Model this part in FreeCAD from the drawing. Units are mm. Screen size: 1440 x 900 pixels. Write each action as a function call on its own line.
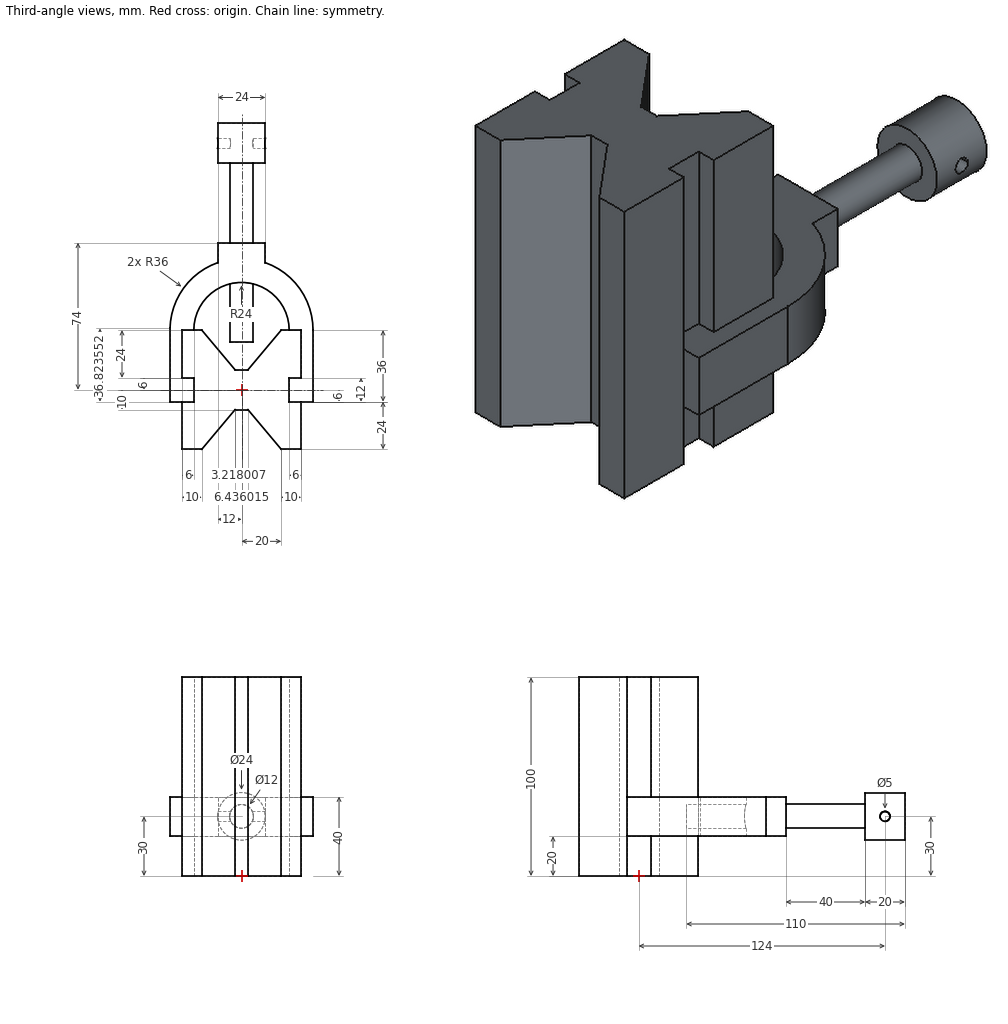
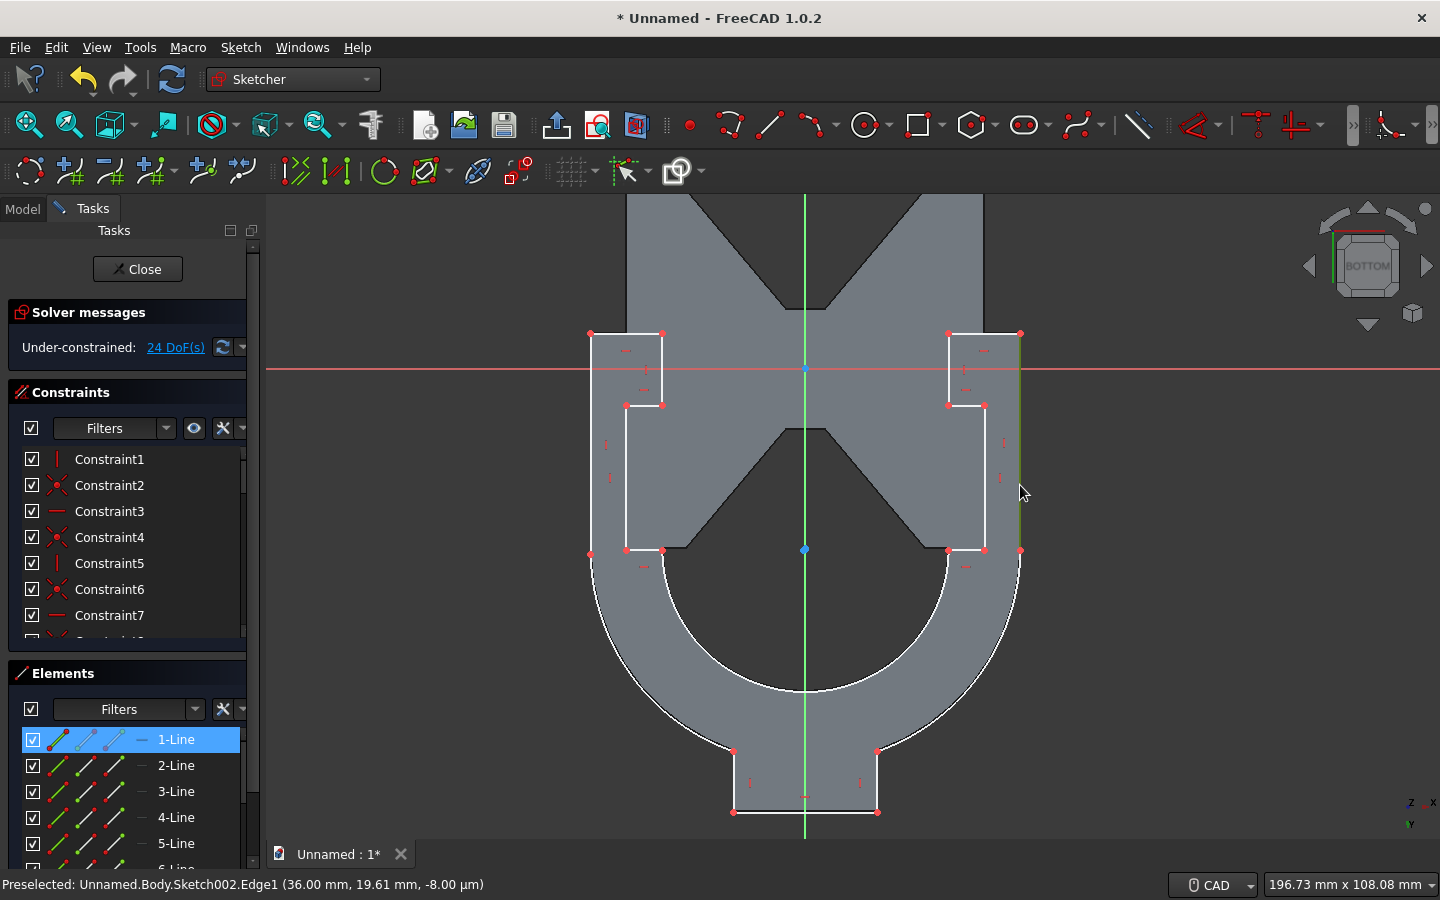
click(945, 712)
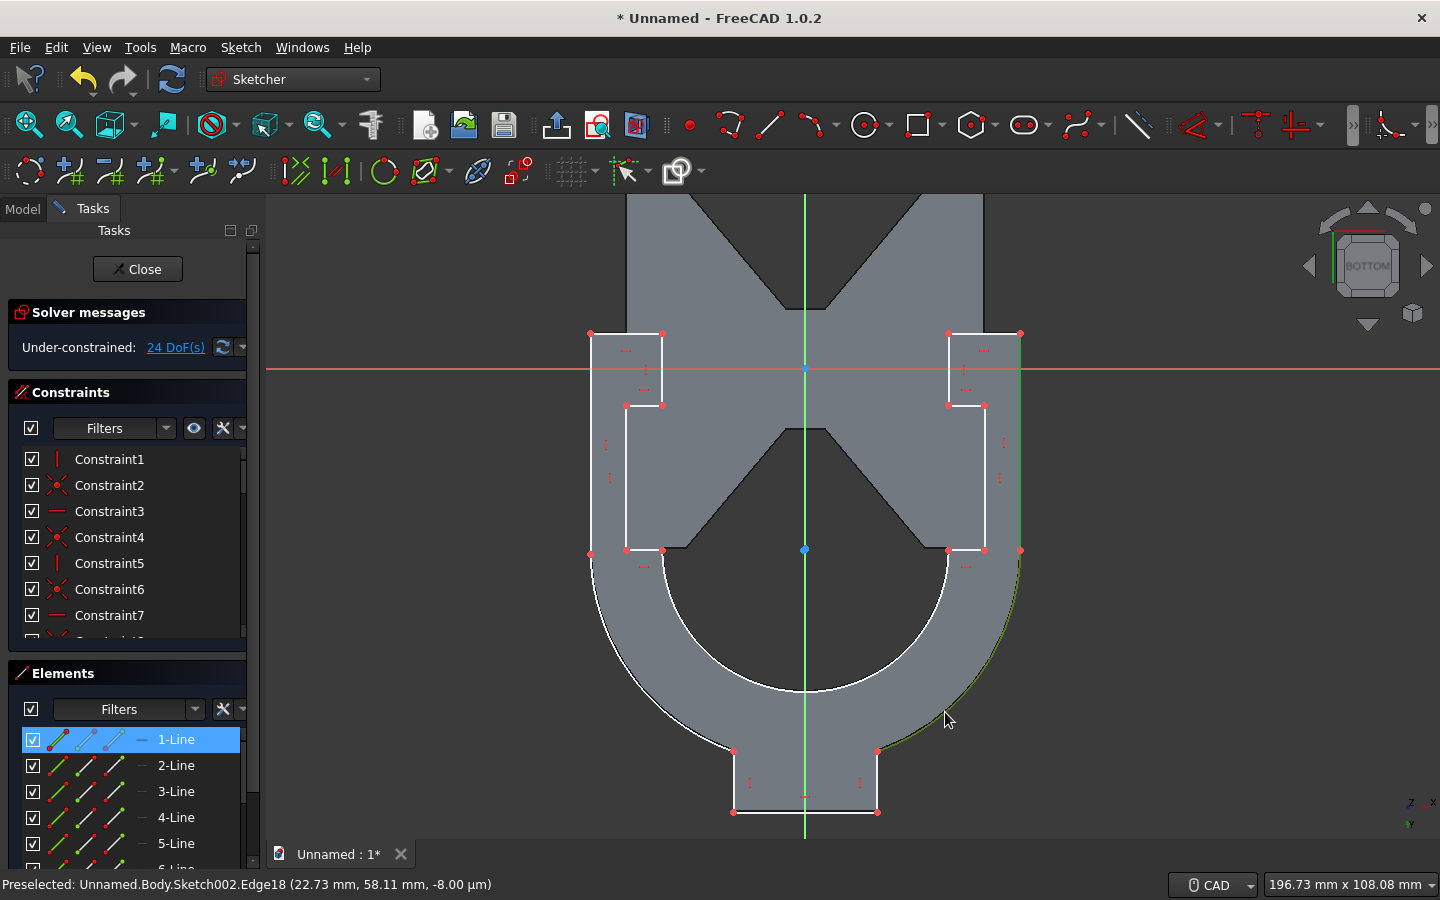
key(t)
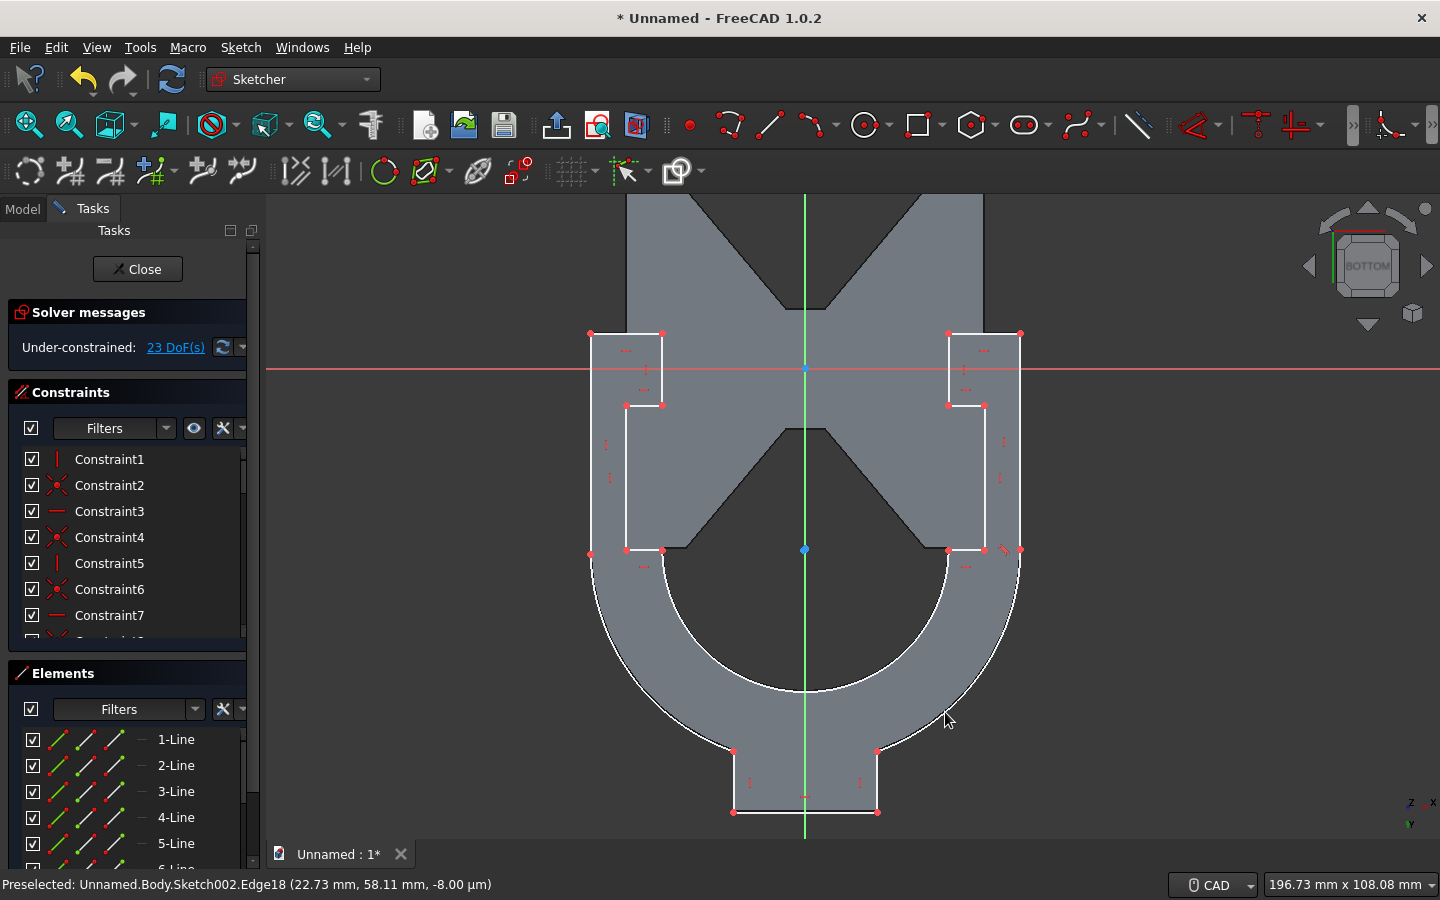
click(722, 665)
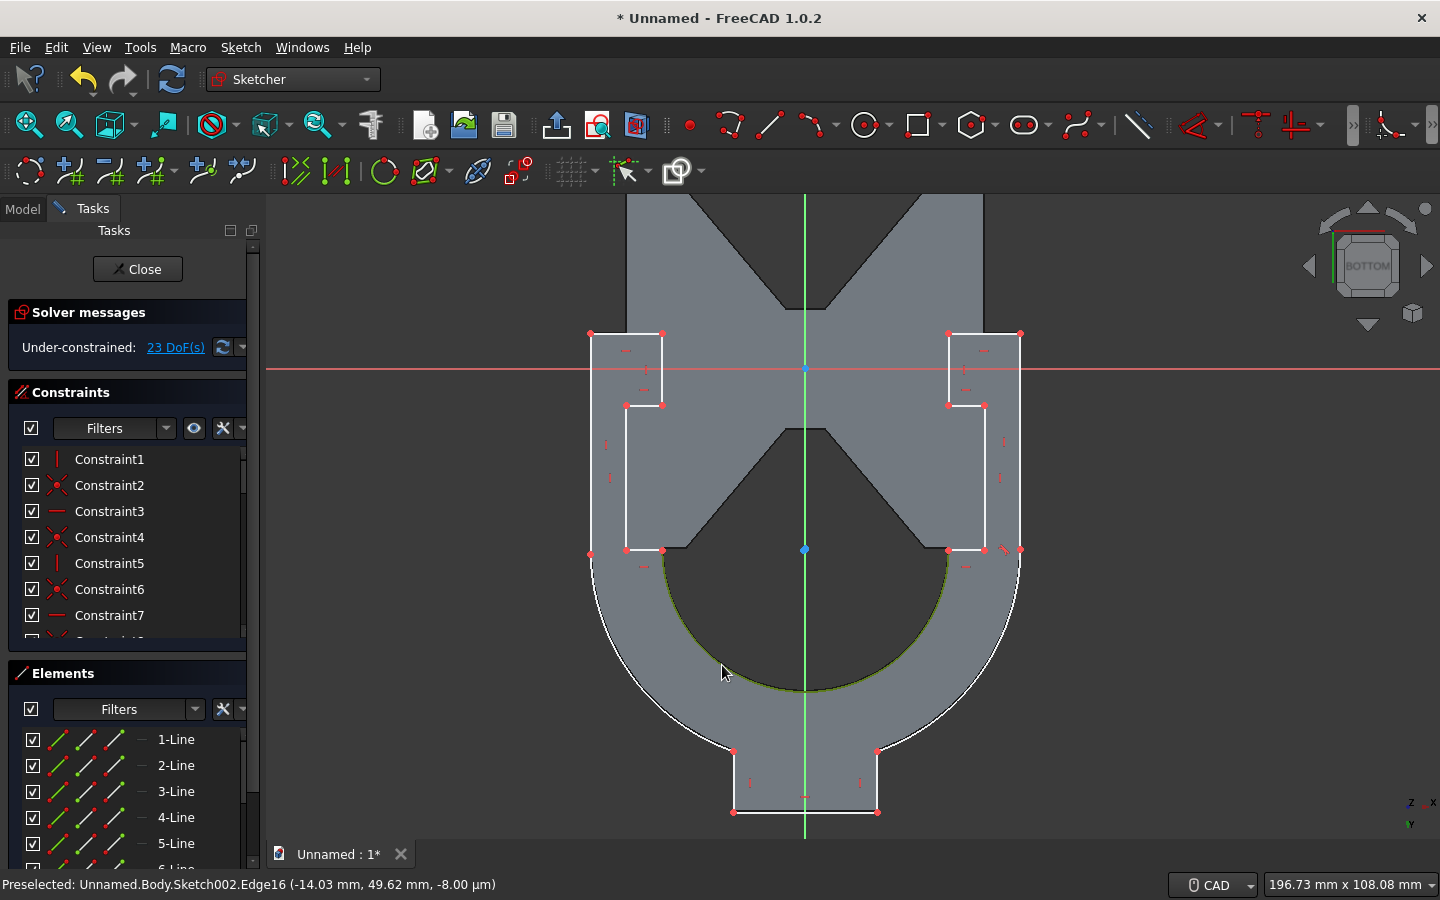
click(606, 630)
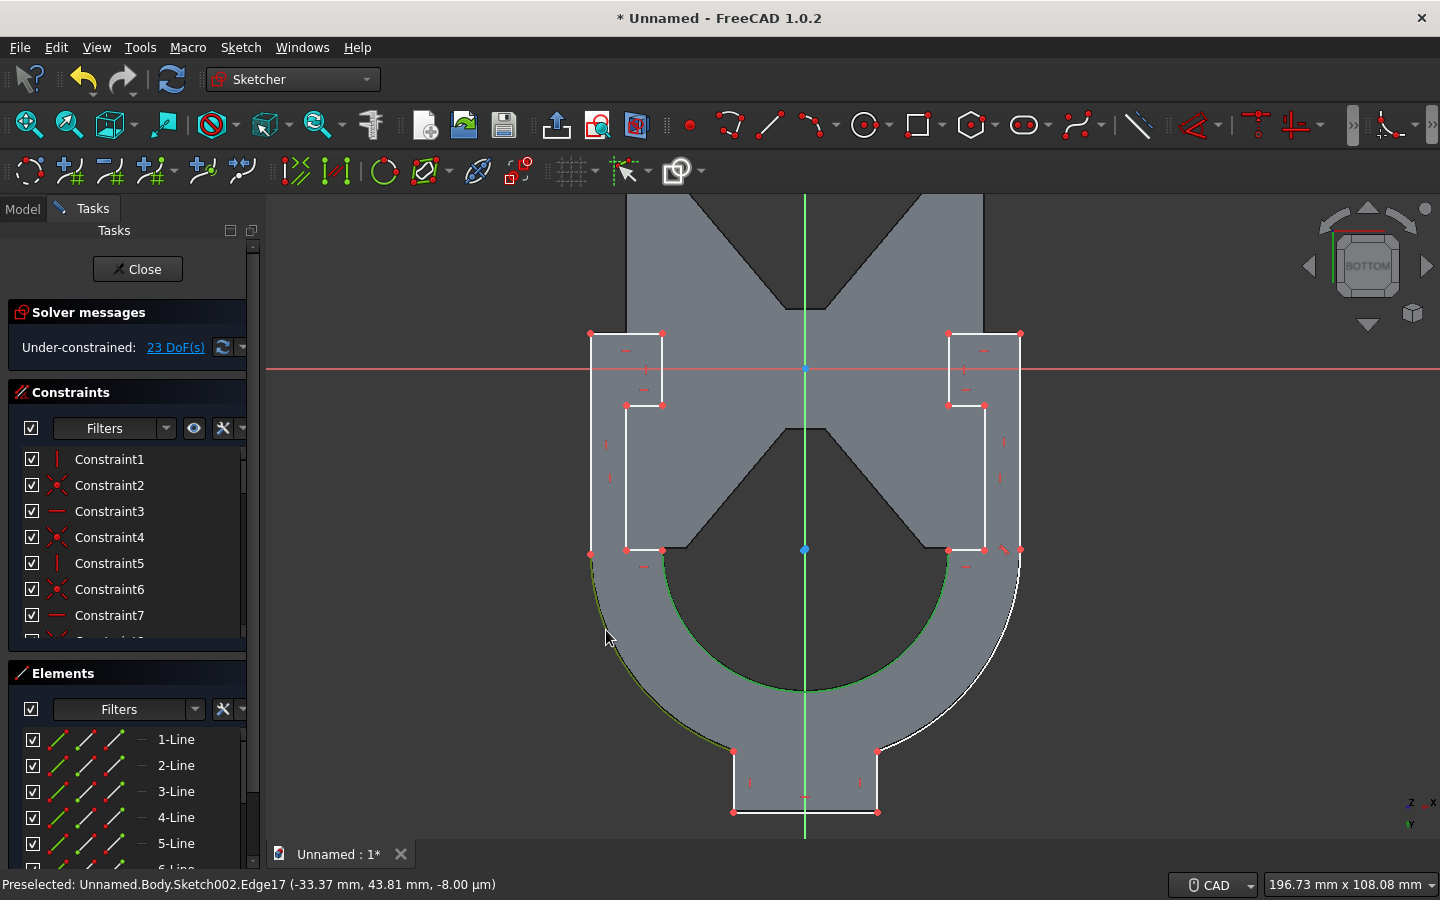
click(1256, 126)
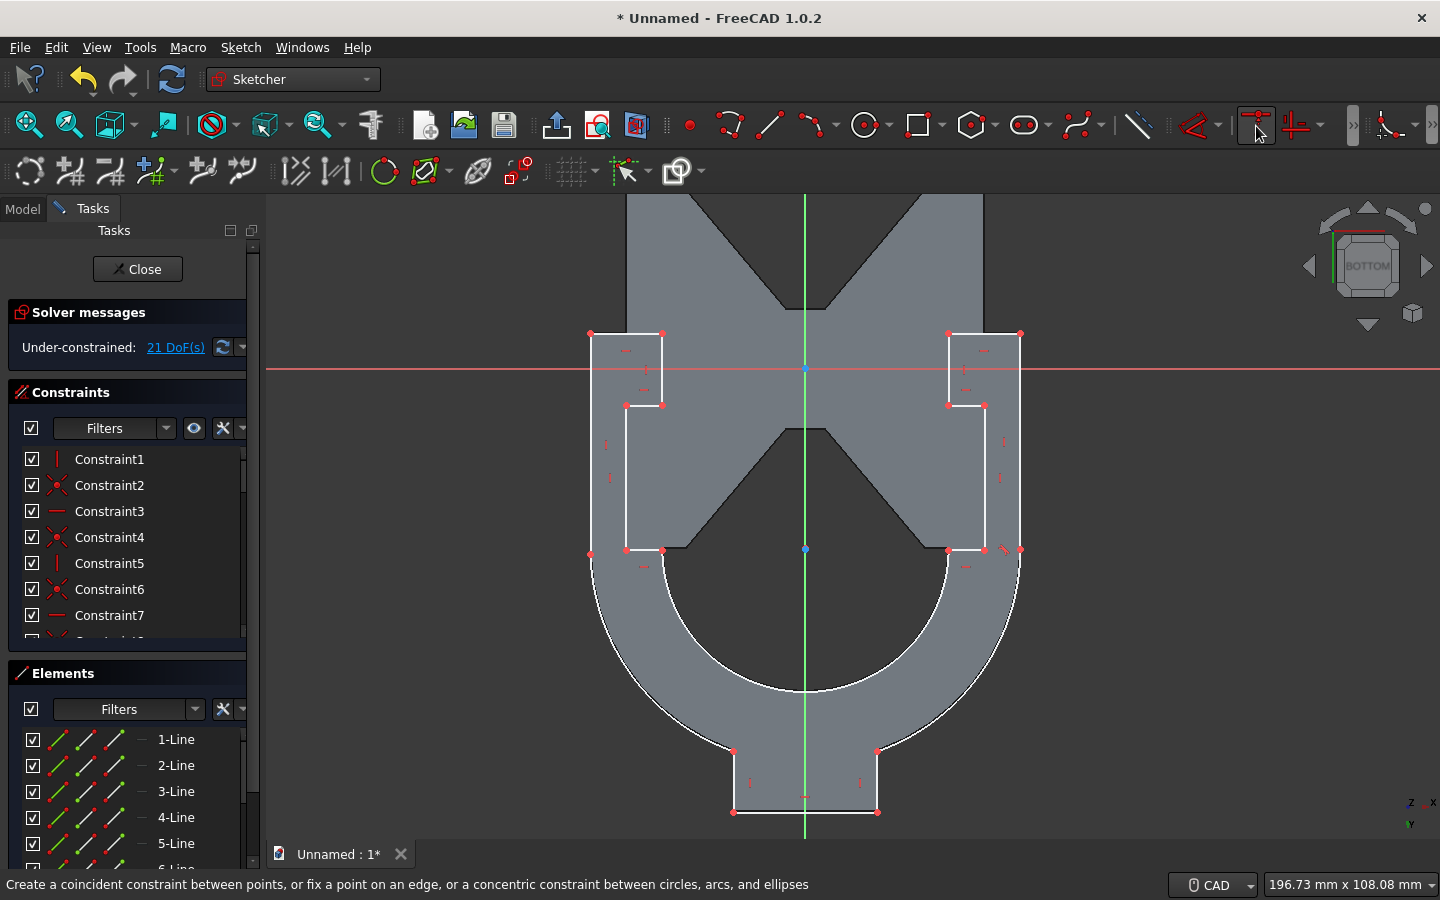
click(722, 665)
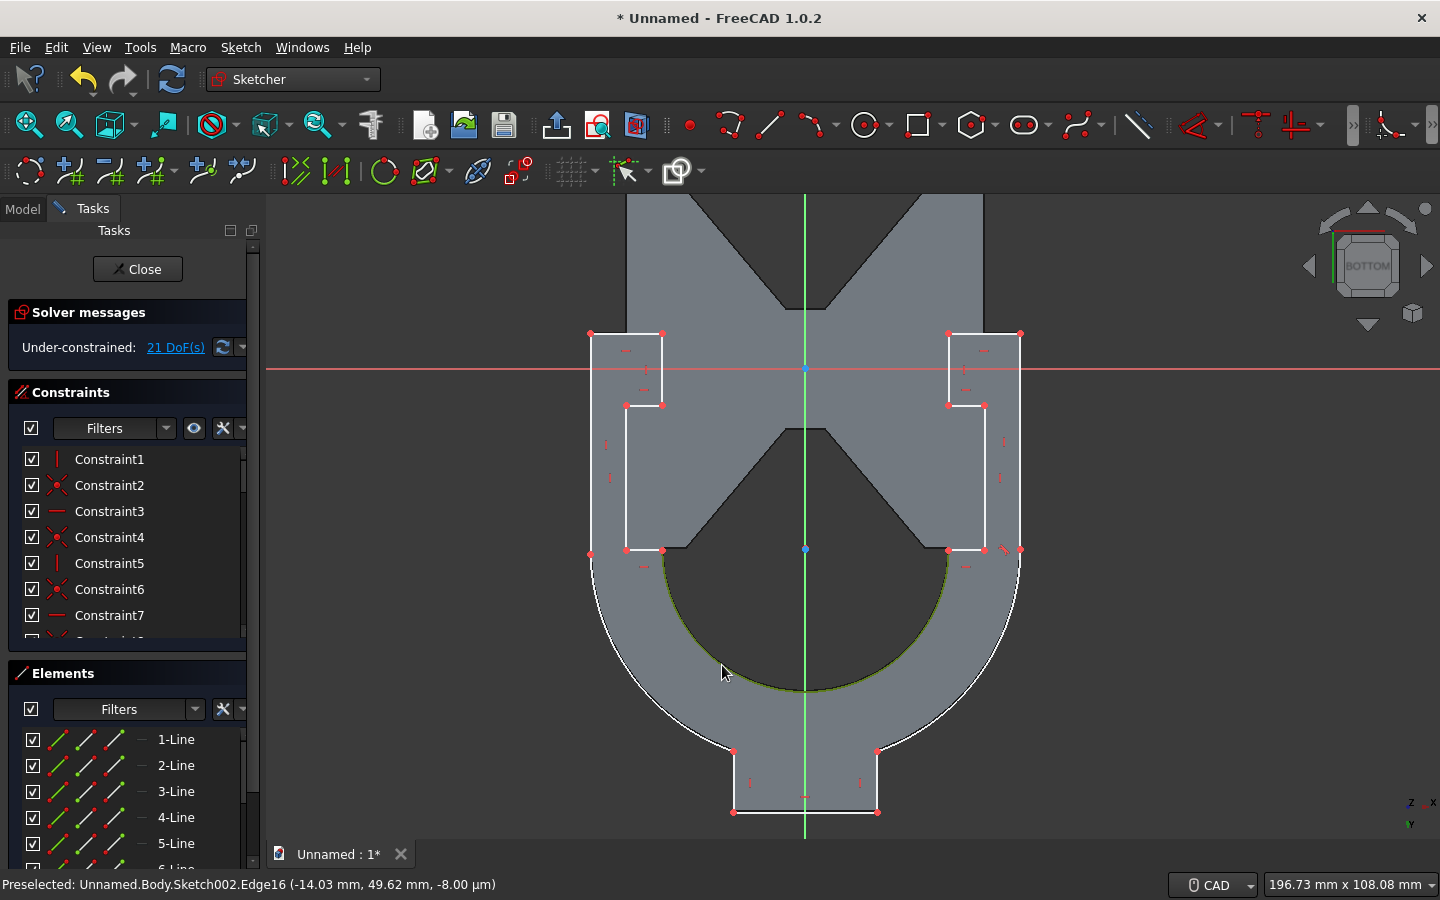
click(945, 712)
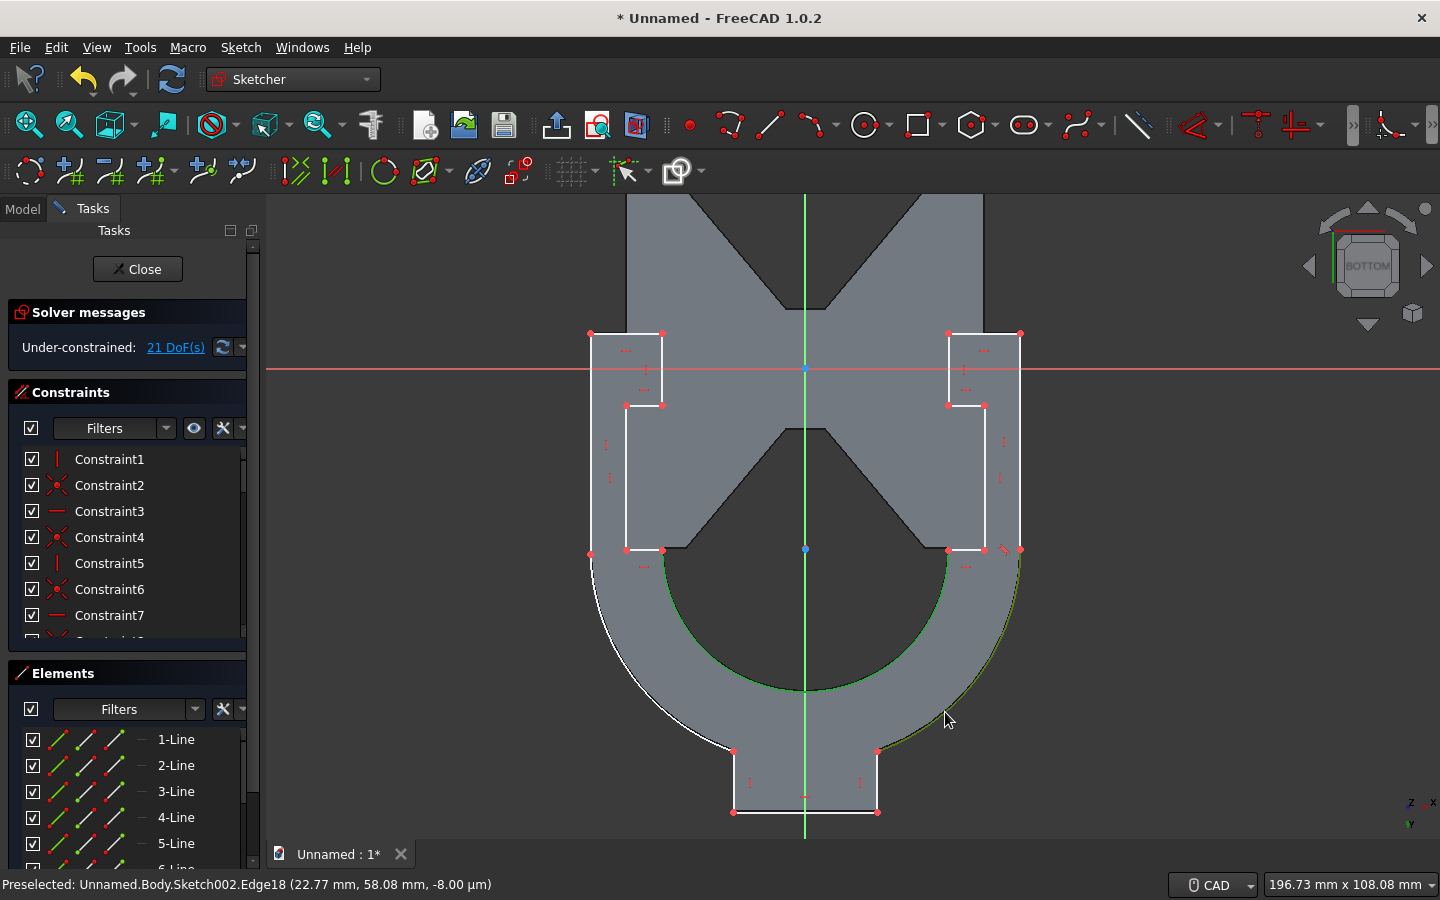
key(c)